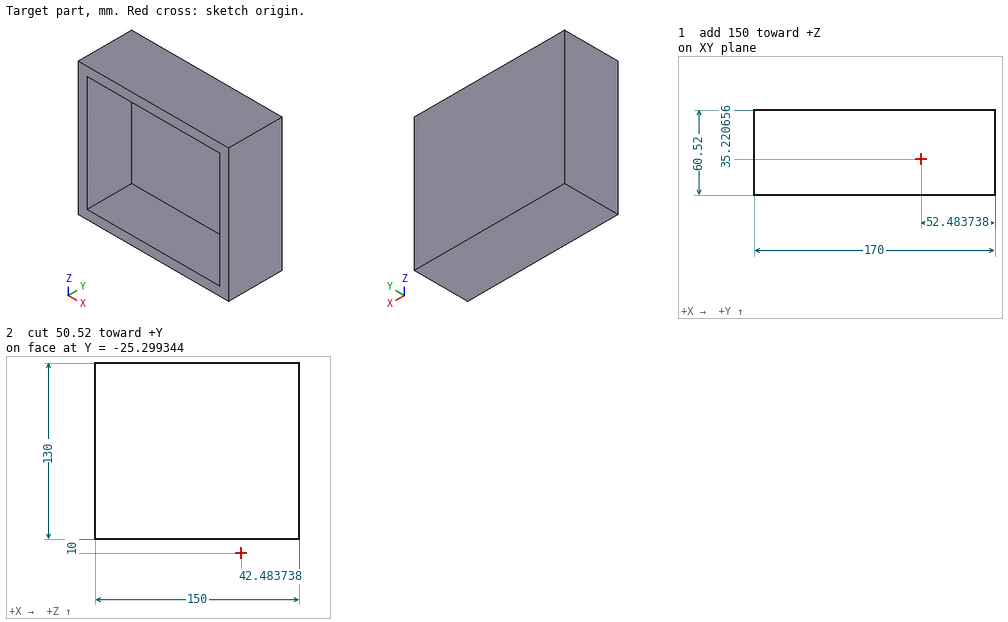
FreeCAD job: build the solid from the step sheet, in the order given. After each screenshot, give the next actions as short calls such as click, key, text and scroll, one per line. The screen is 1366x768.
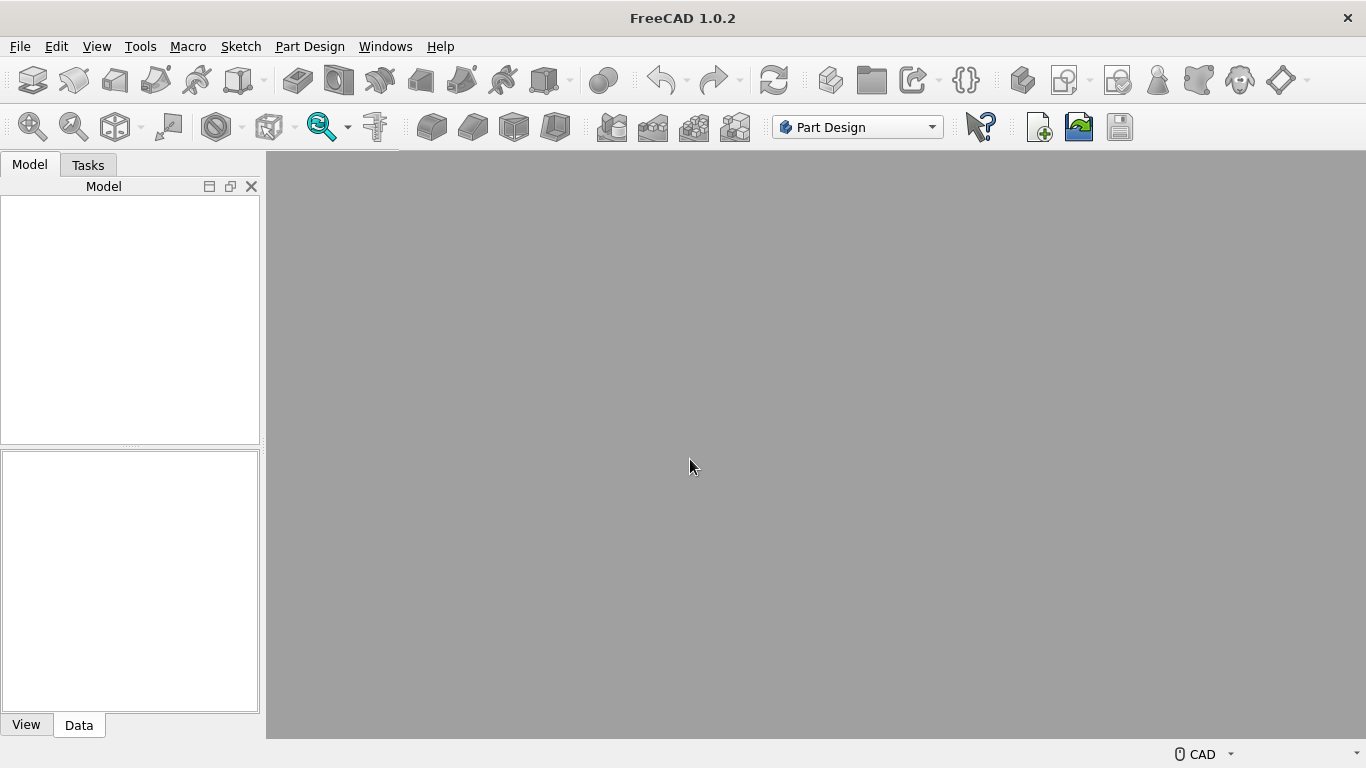
click(1038, 128)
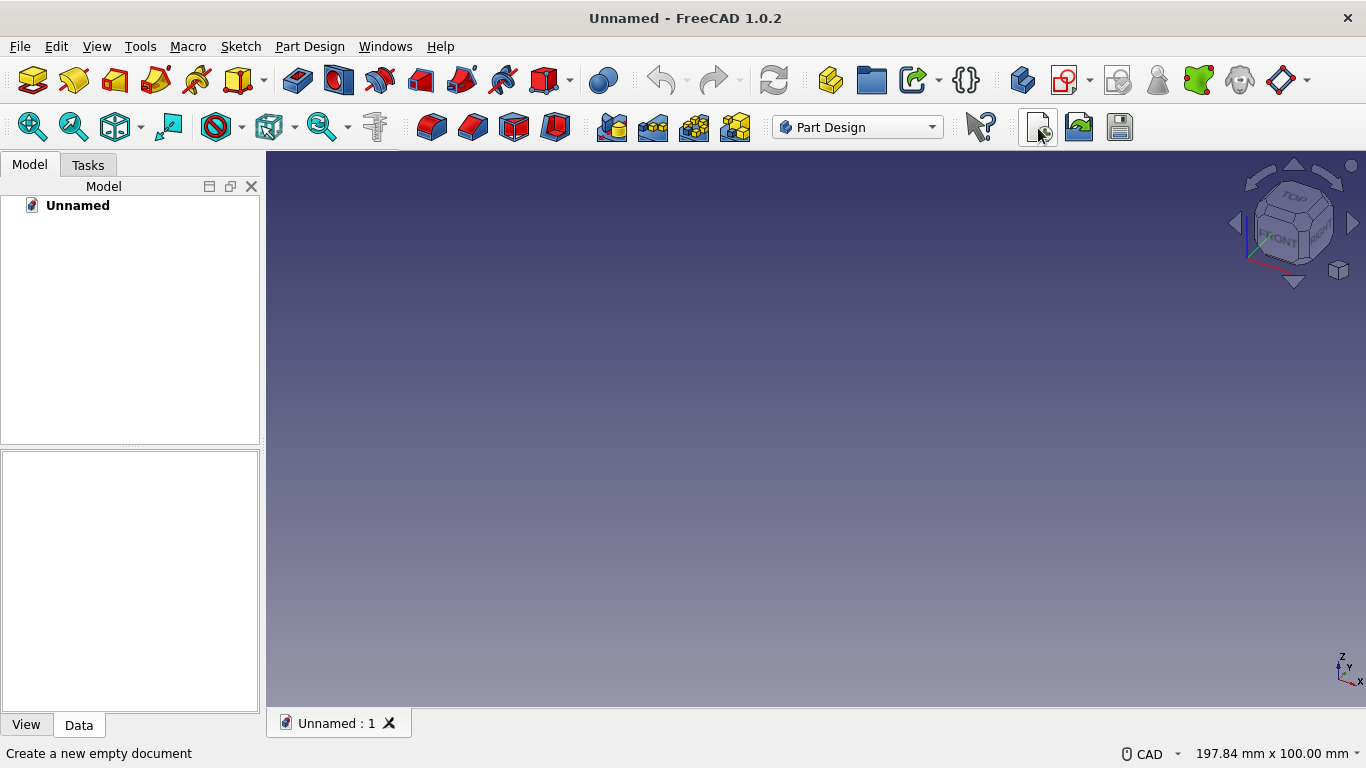
click(1064, 80)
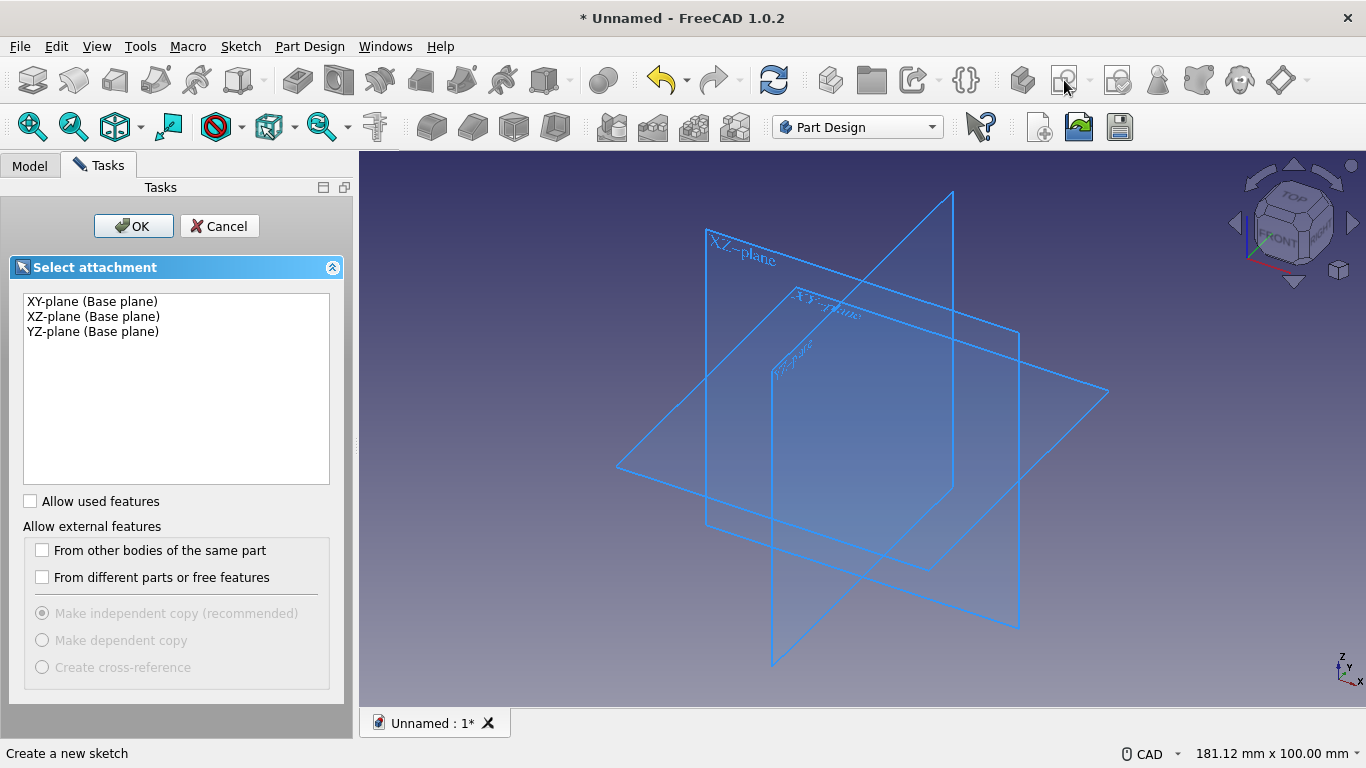
click(84, 302)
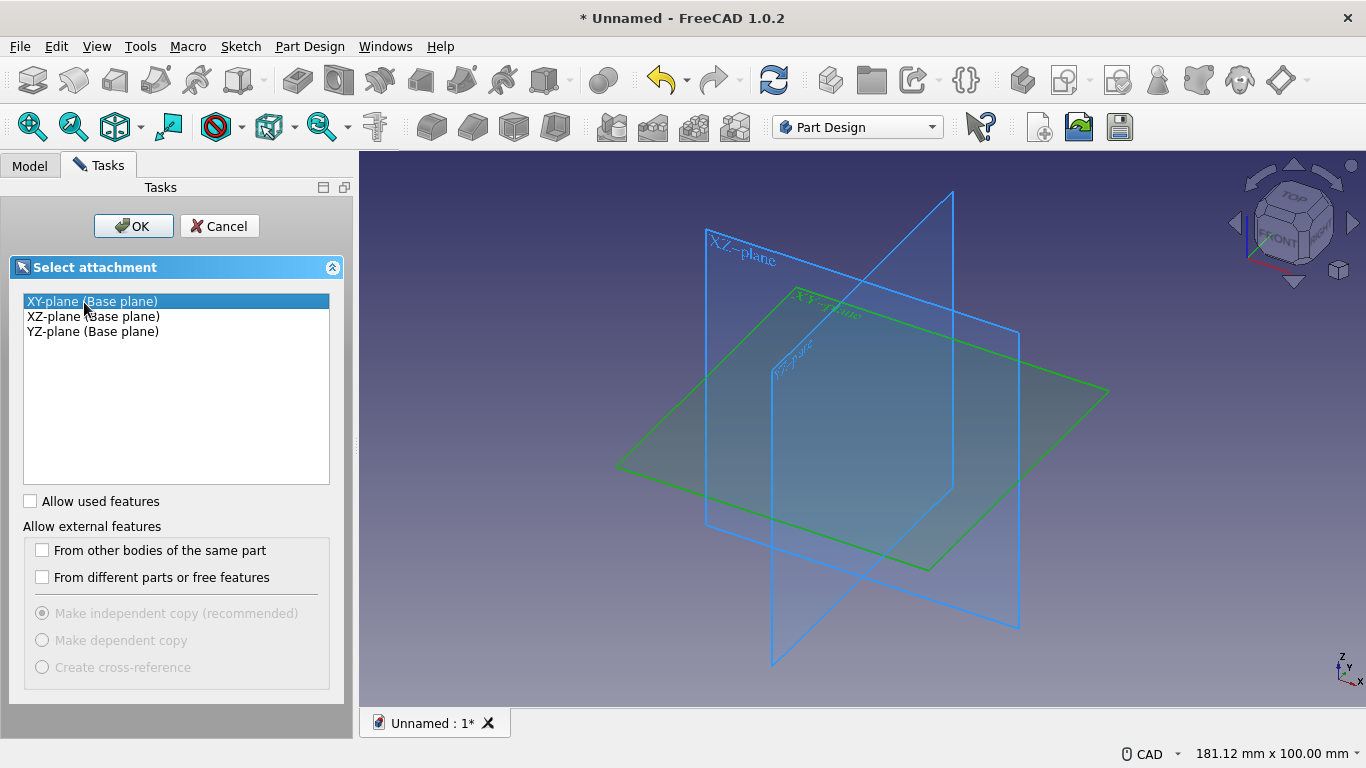
click(134, 226)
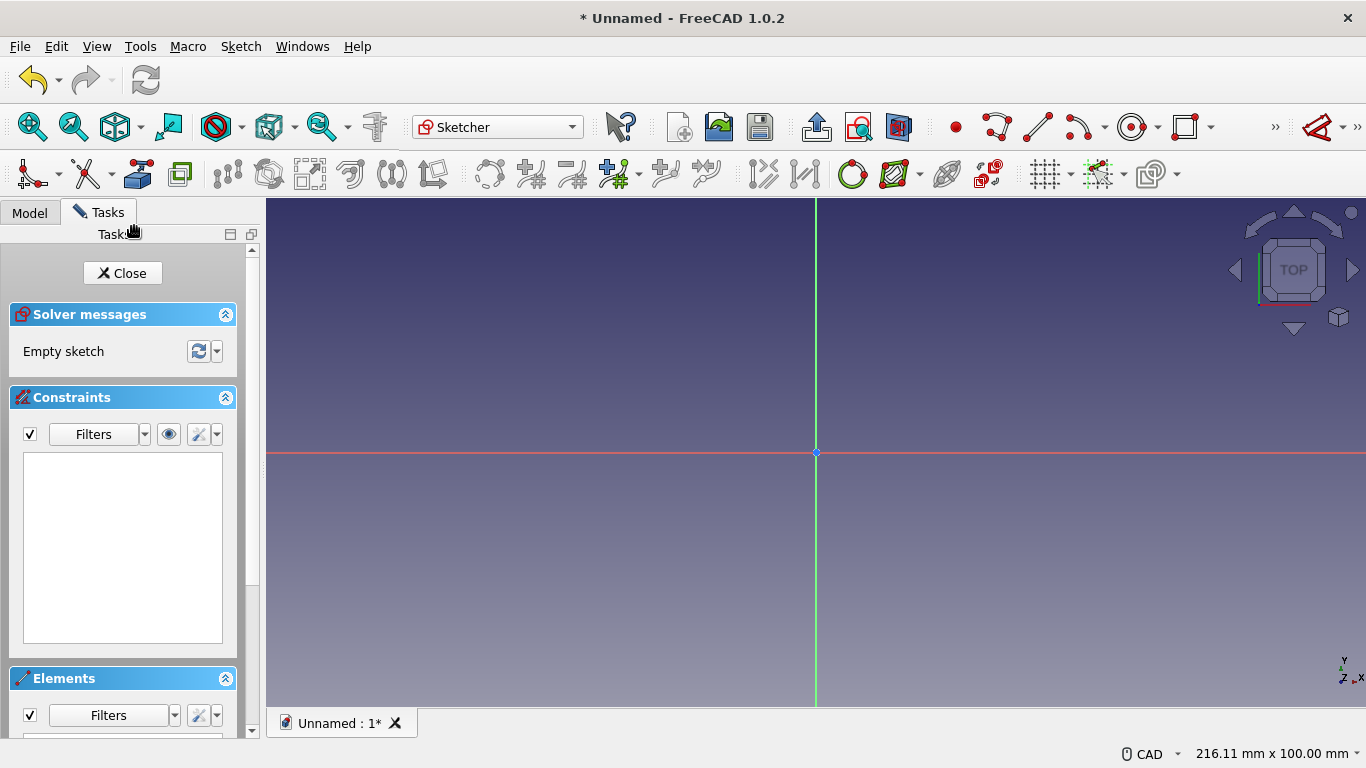
scroll(945, 504, down, 2)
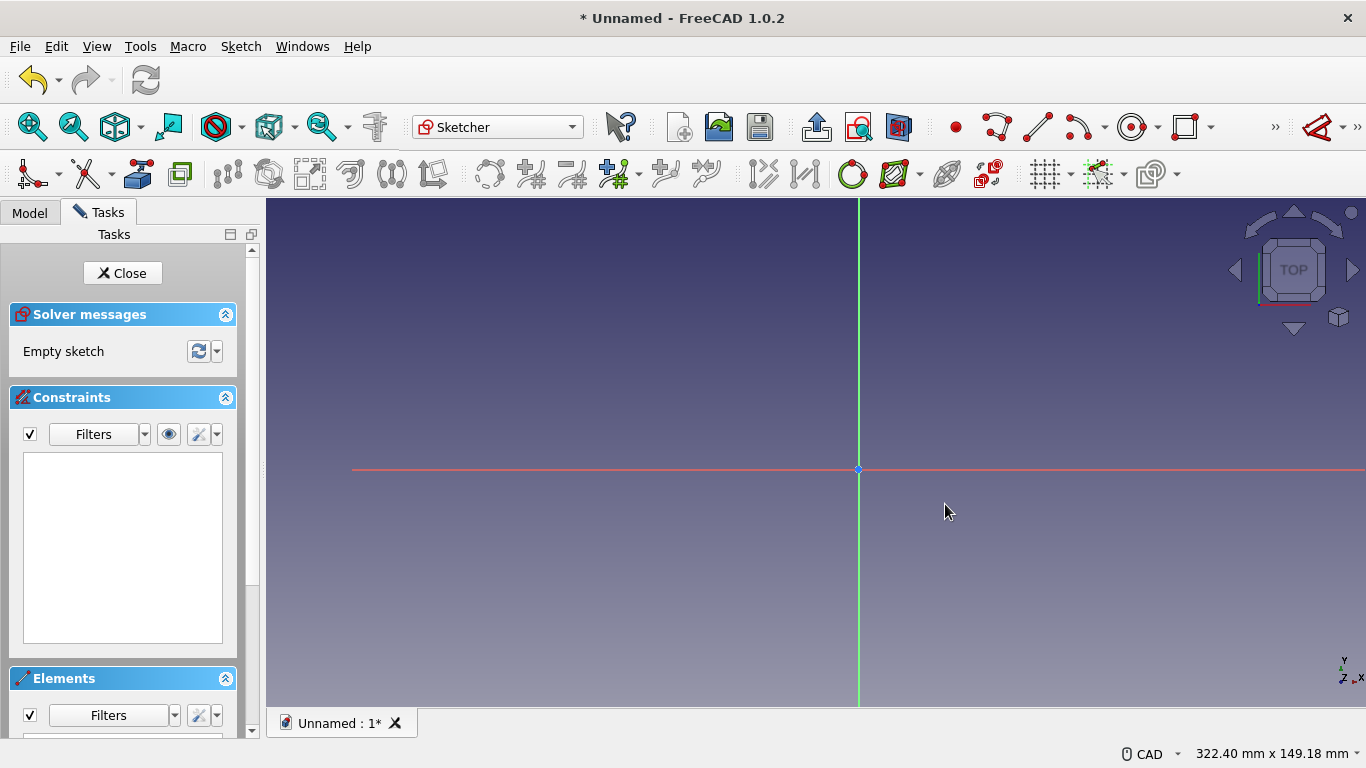
click(1184, 128)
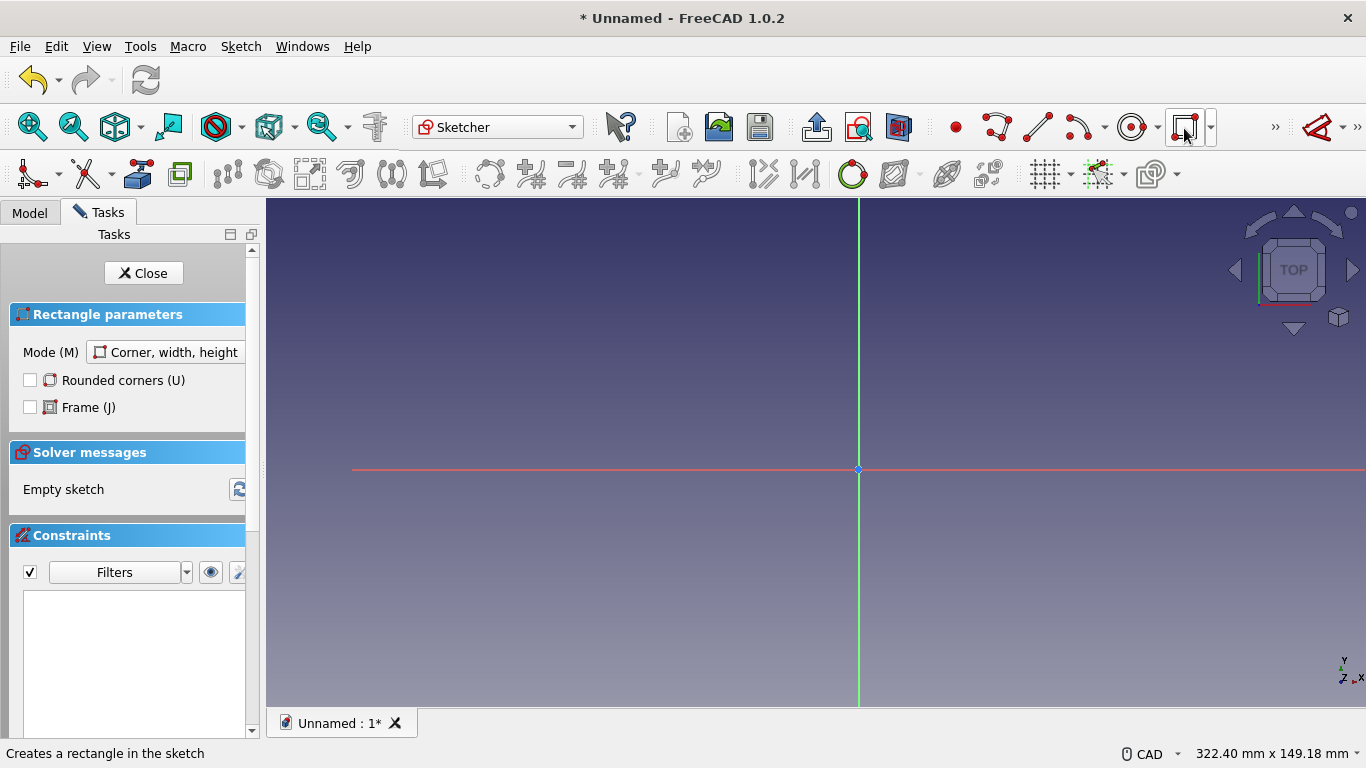
click(458, 350)
click(1038, 556)
key(Escape)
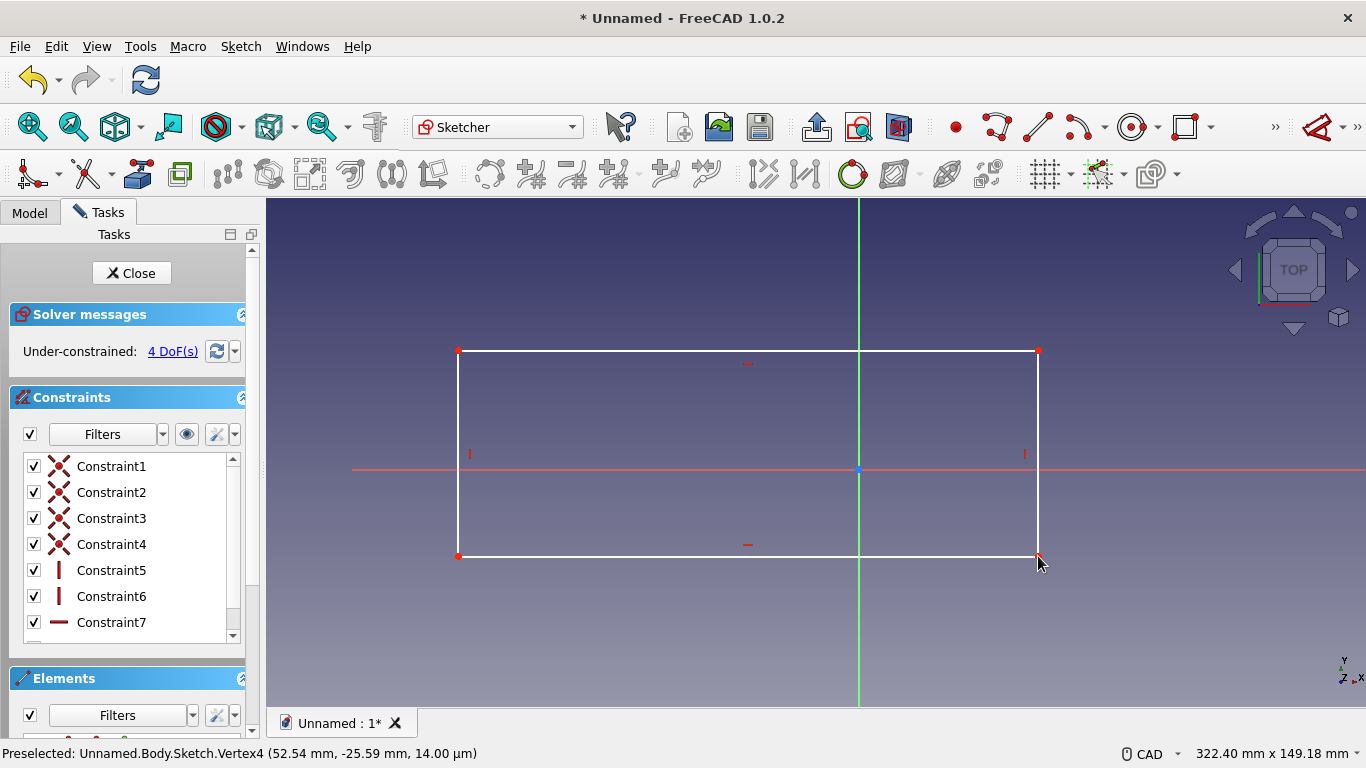
click(632, 557)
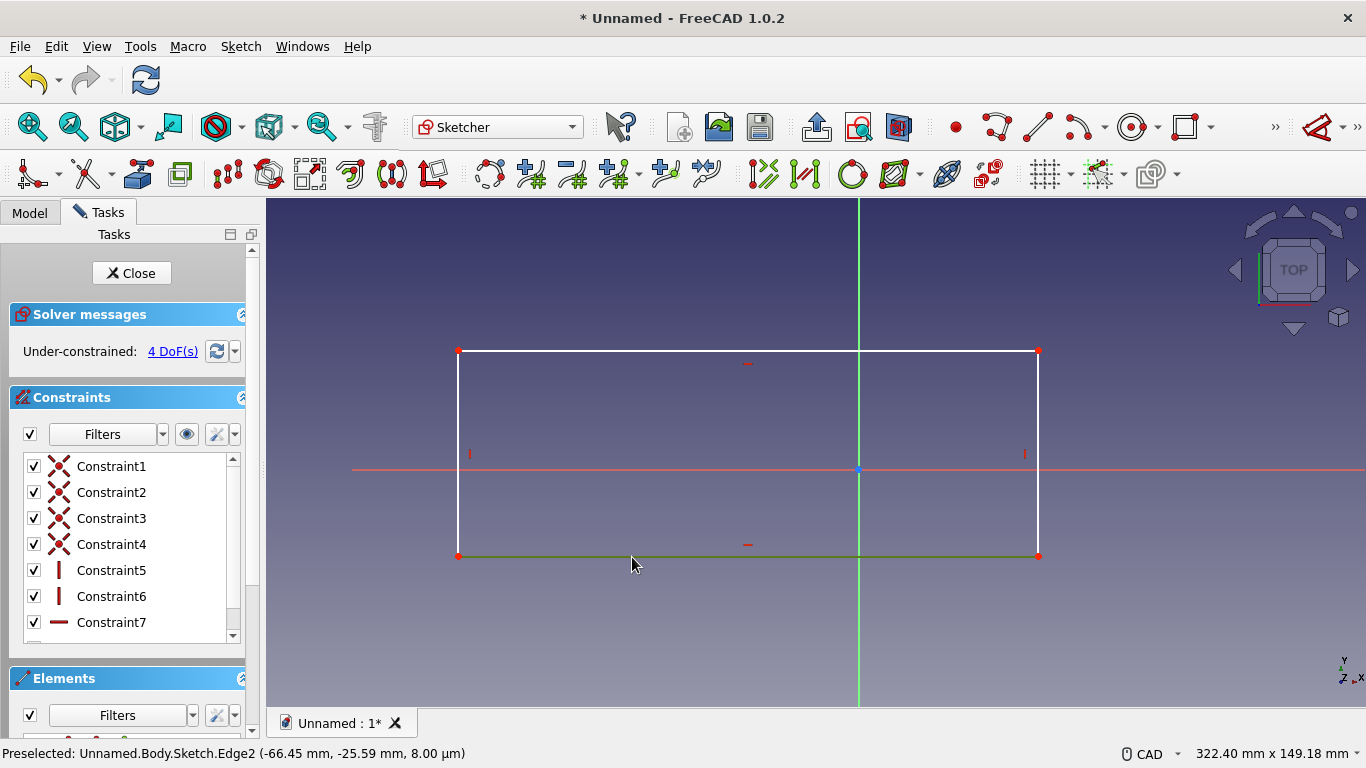
click(1342, 128)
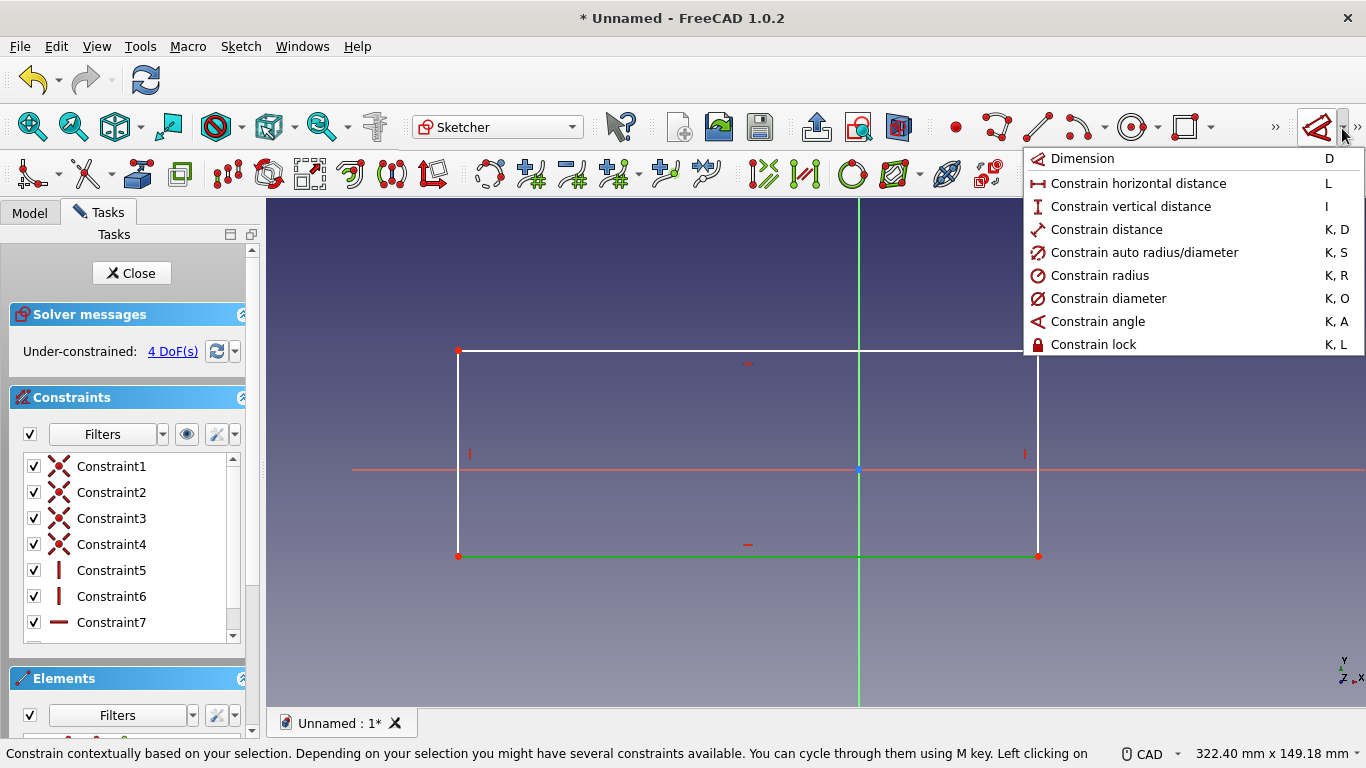
click(1194, 184)